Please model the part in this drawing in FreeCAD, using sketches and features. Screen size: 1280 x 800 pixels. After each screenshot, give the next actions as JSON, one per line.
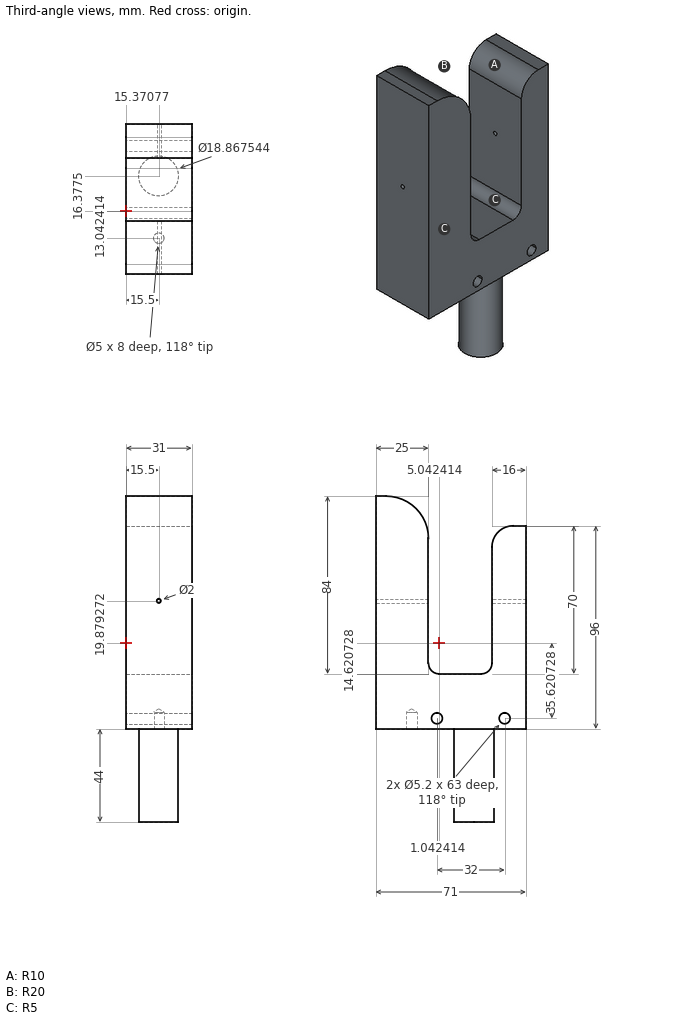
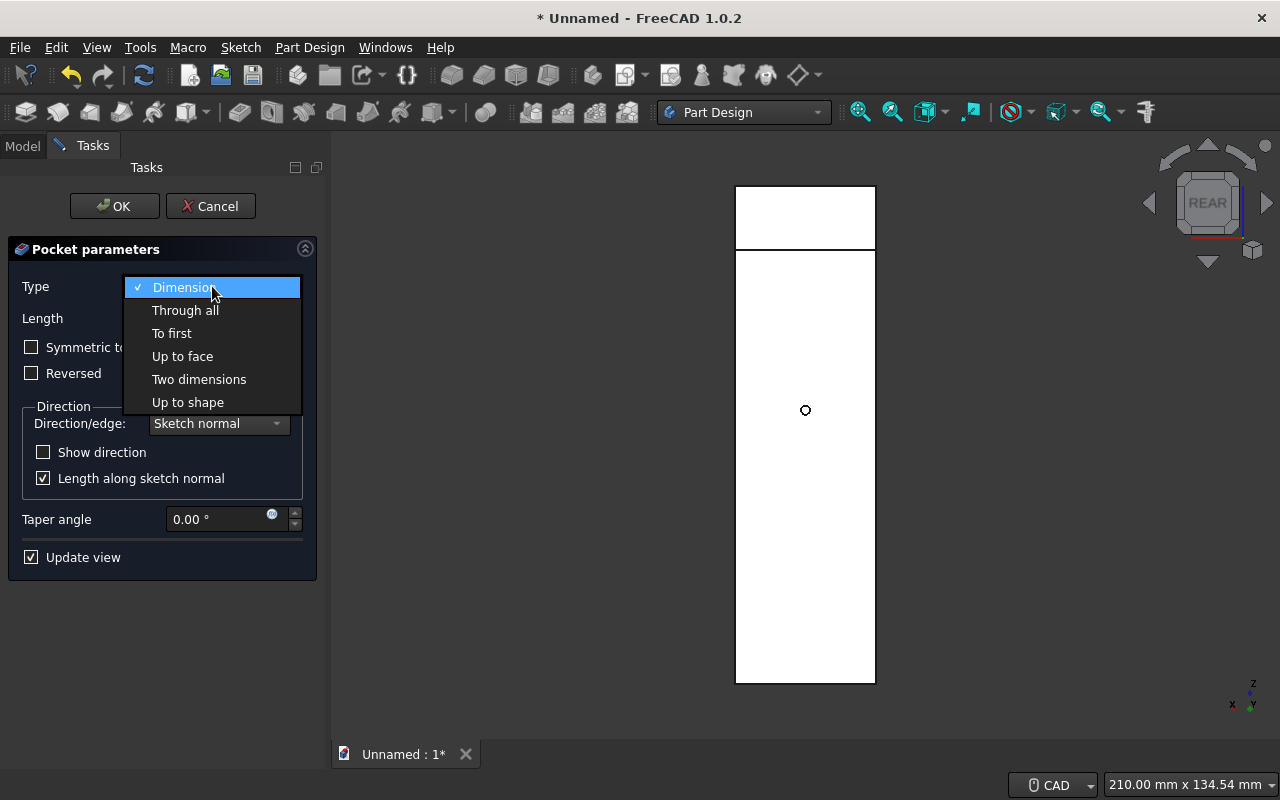
{"action": "left_click", "coordinate": [212, 310]}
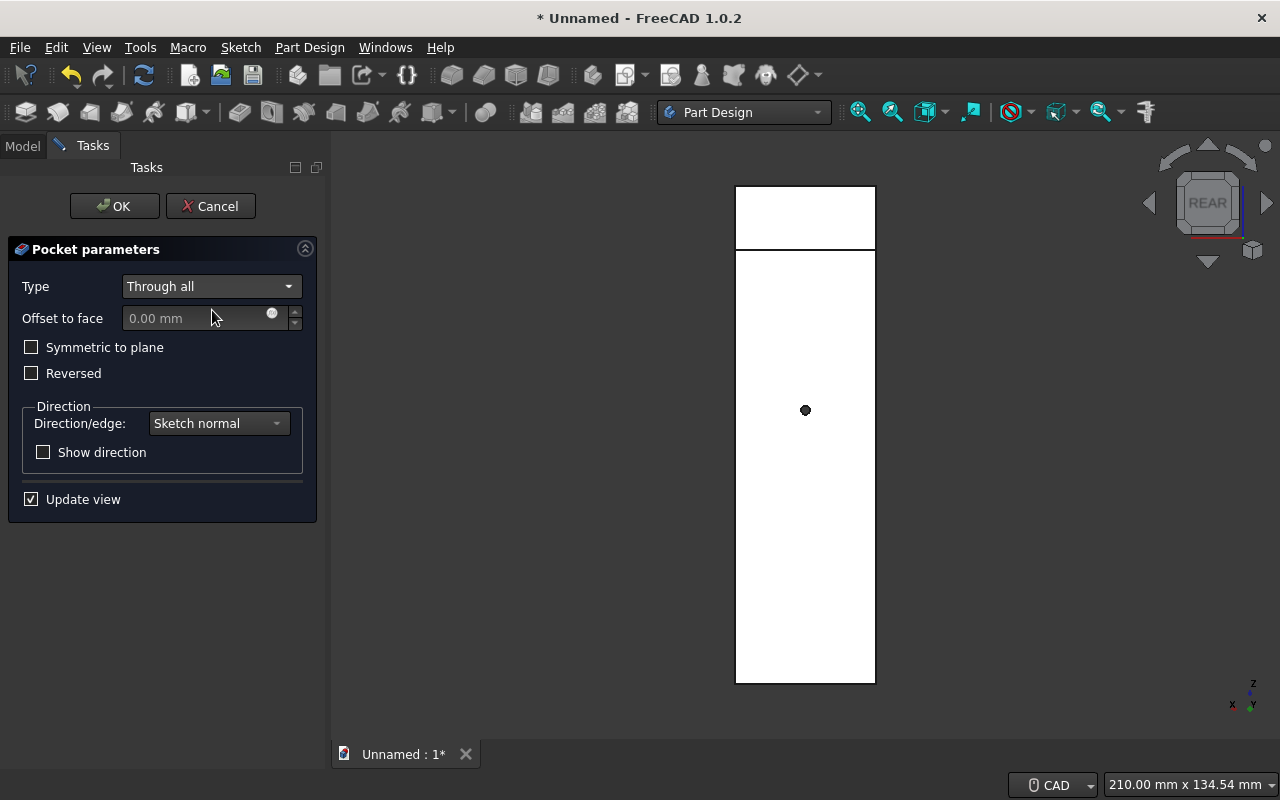
{"action": "left_click", "coordinate": [115, 206]}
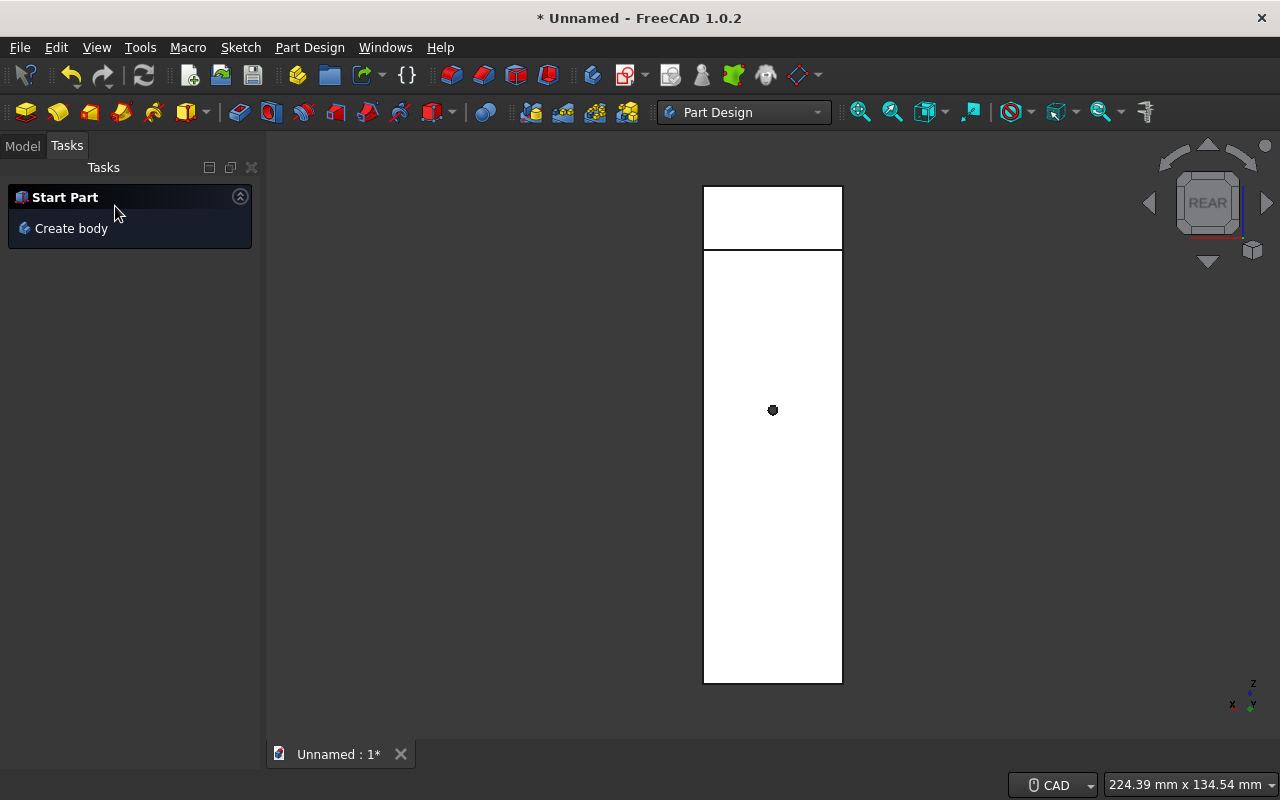
{"action": "key", "text": "0"}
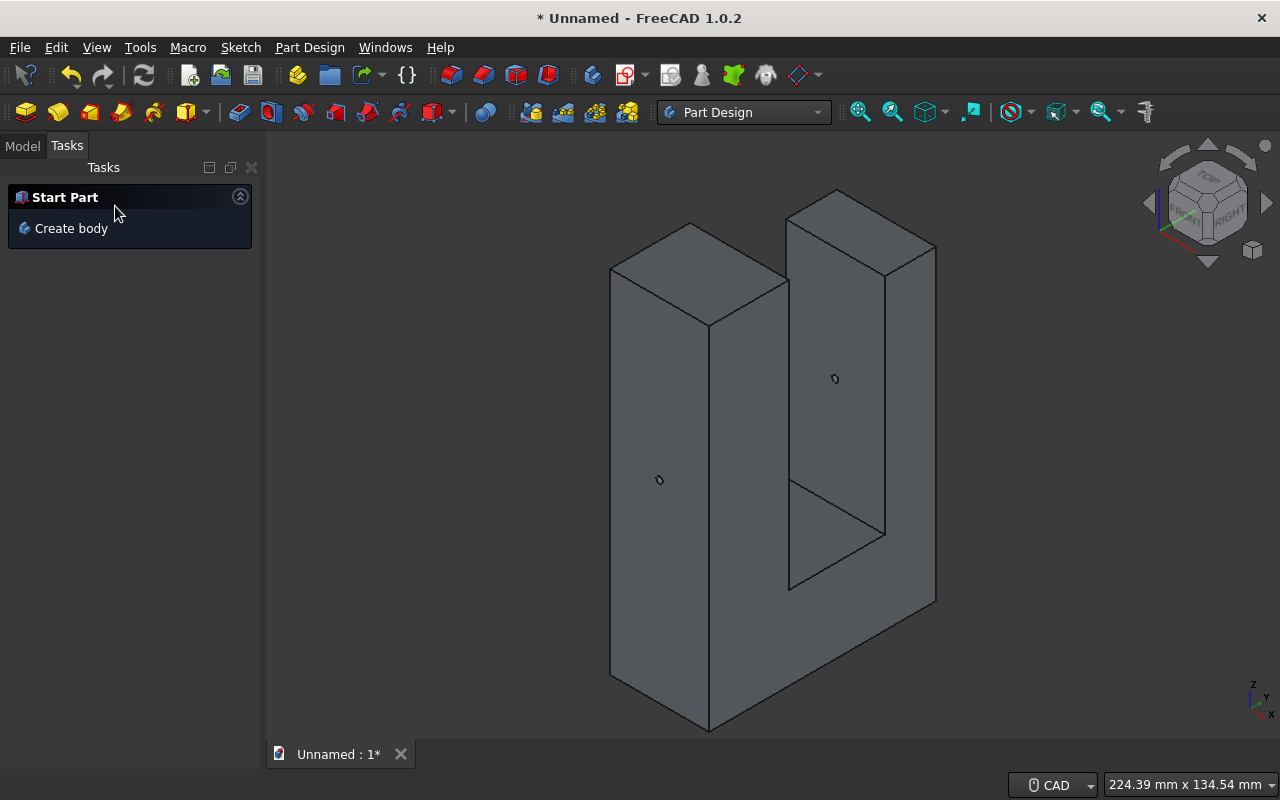
{"action": "left_click", "coordinate": [835, 247]}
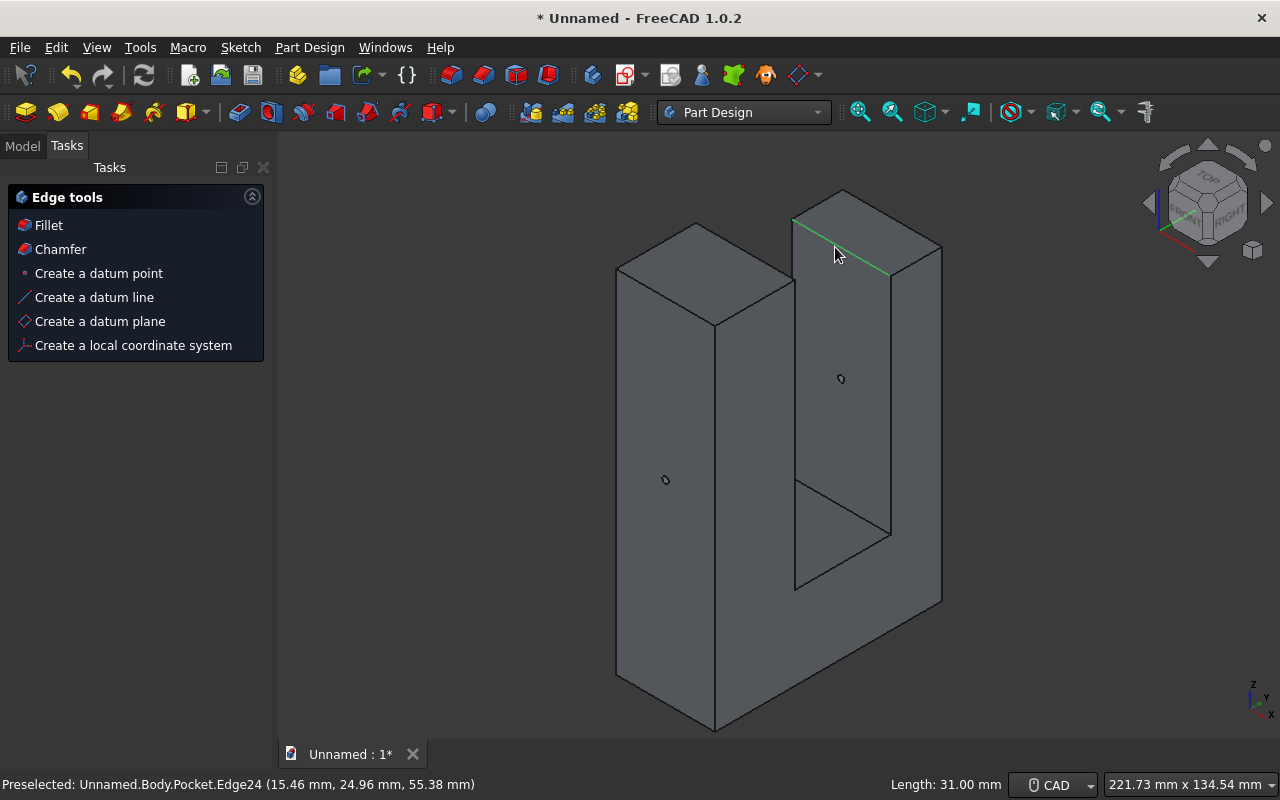
{"action": "left_click", "coordinate": [452, 76]}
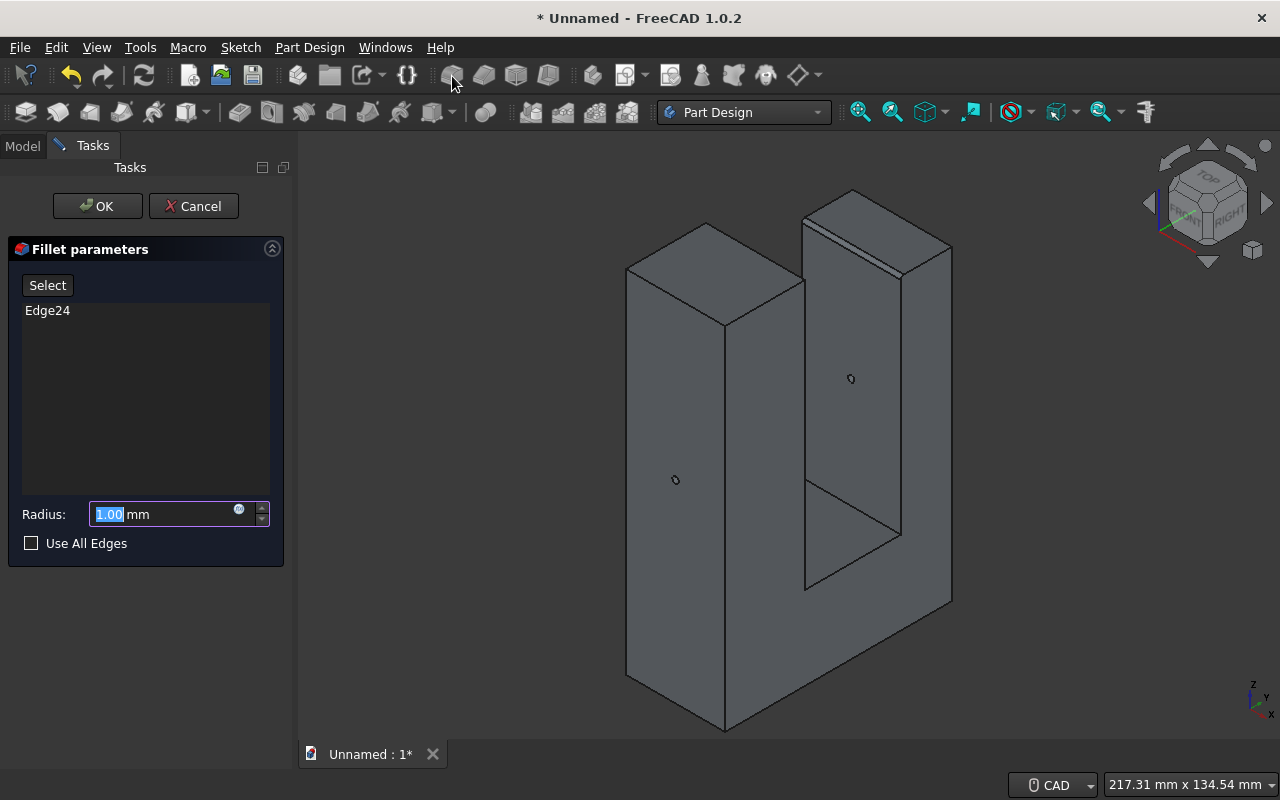
{"action": "type", "text": "10"}
{"action": "key", "text": "Tab"}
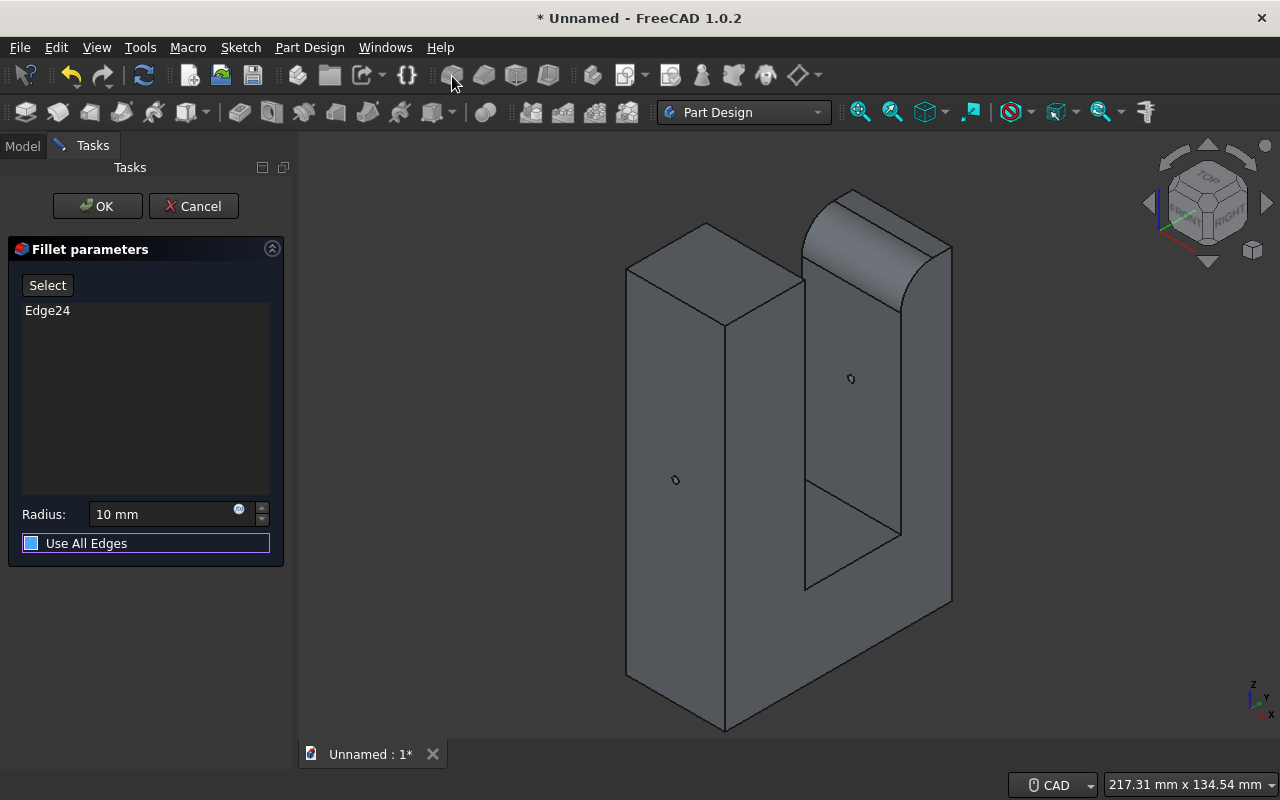
{"action": "left_click", "coordinate": [98, 206]}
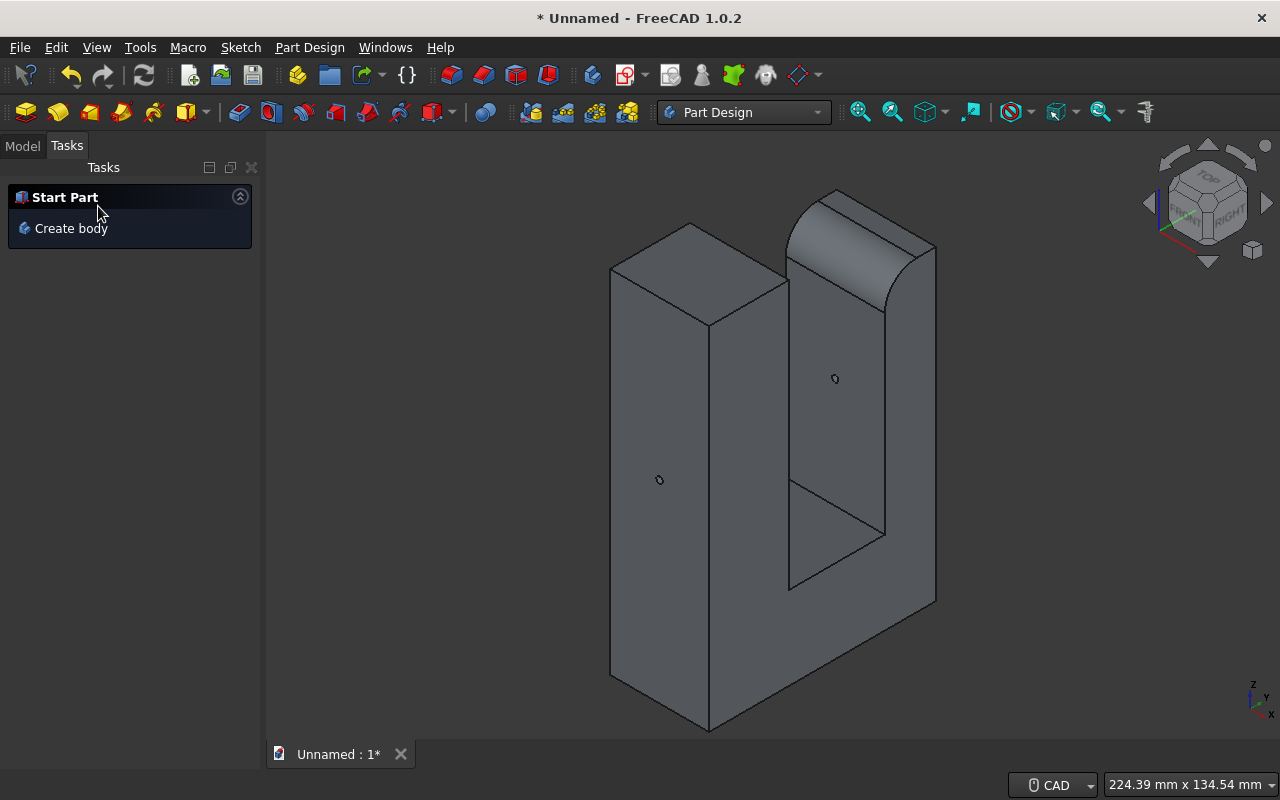
{"action": "key", "text": "2"}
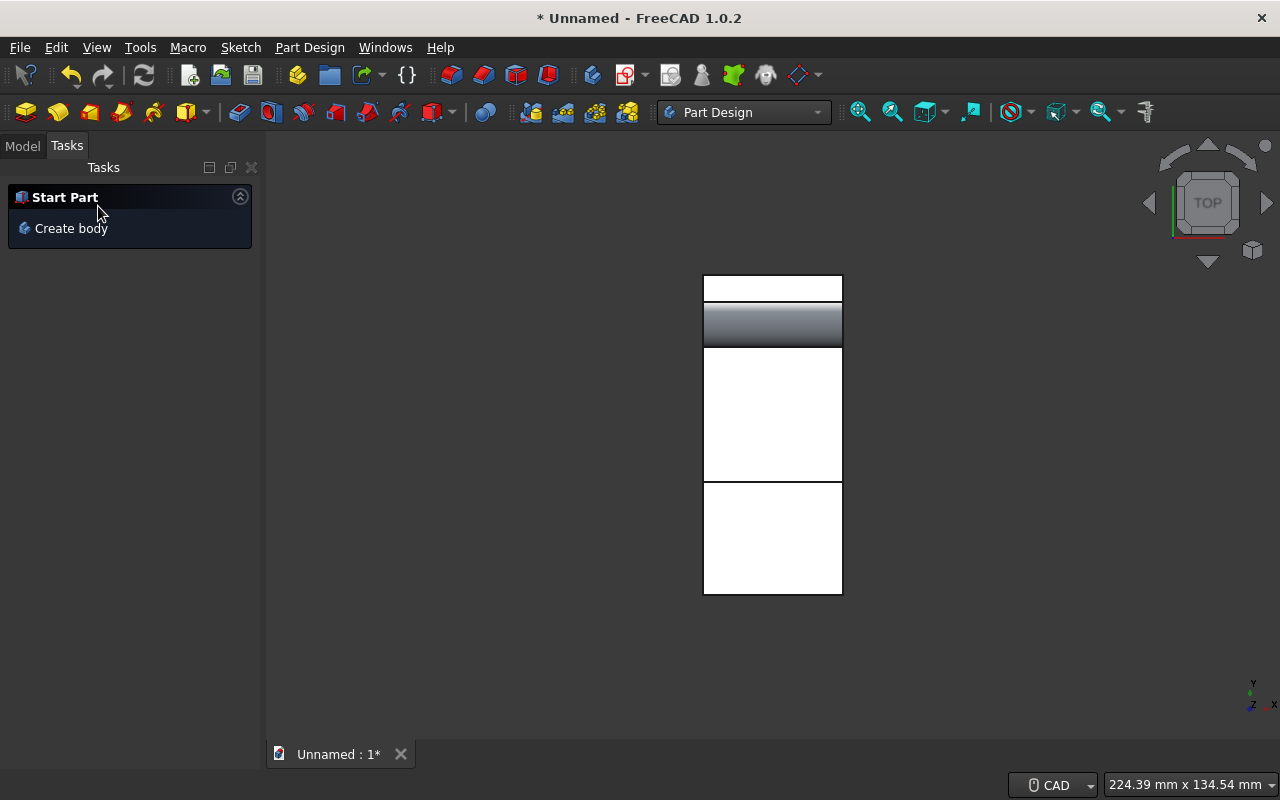
{"action": "left_click", "coordinate": [773, 481]}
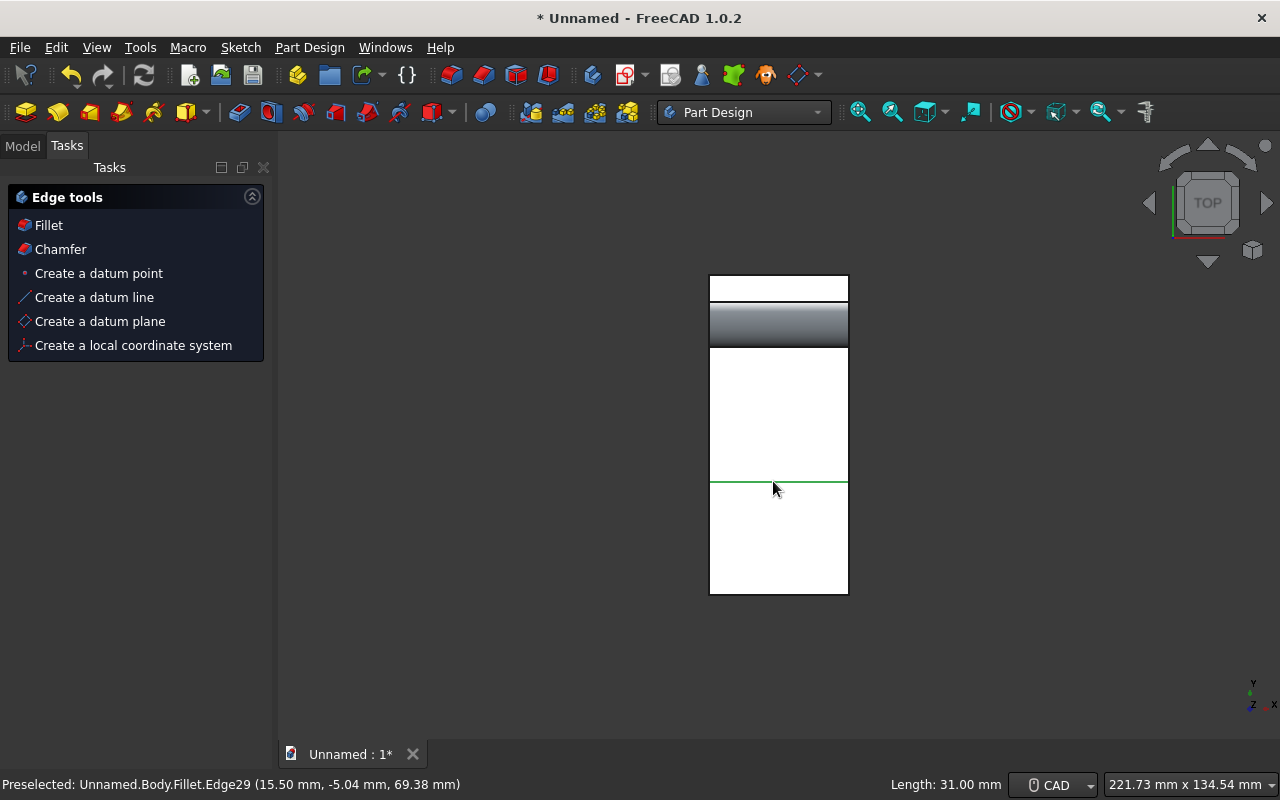
{"action": "left_click", "coordinate": [452, 76]}